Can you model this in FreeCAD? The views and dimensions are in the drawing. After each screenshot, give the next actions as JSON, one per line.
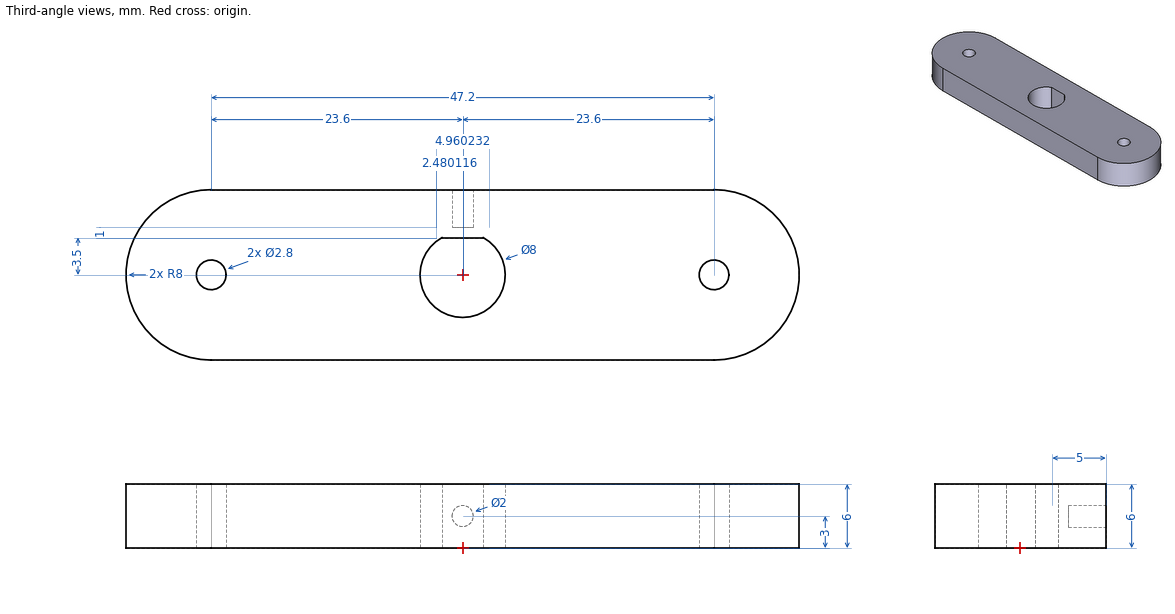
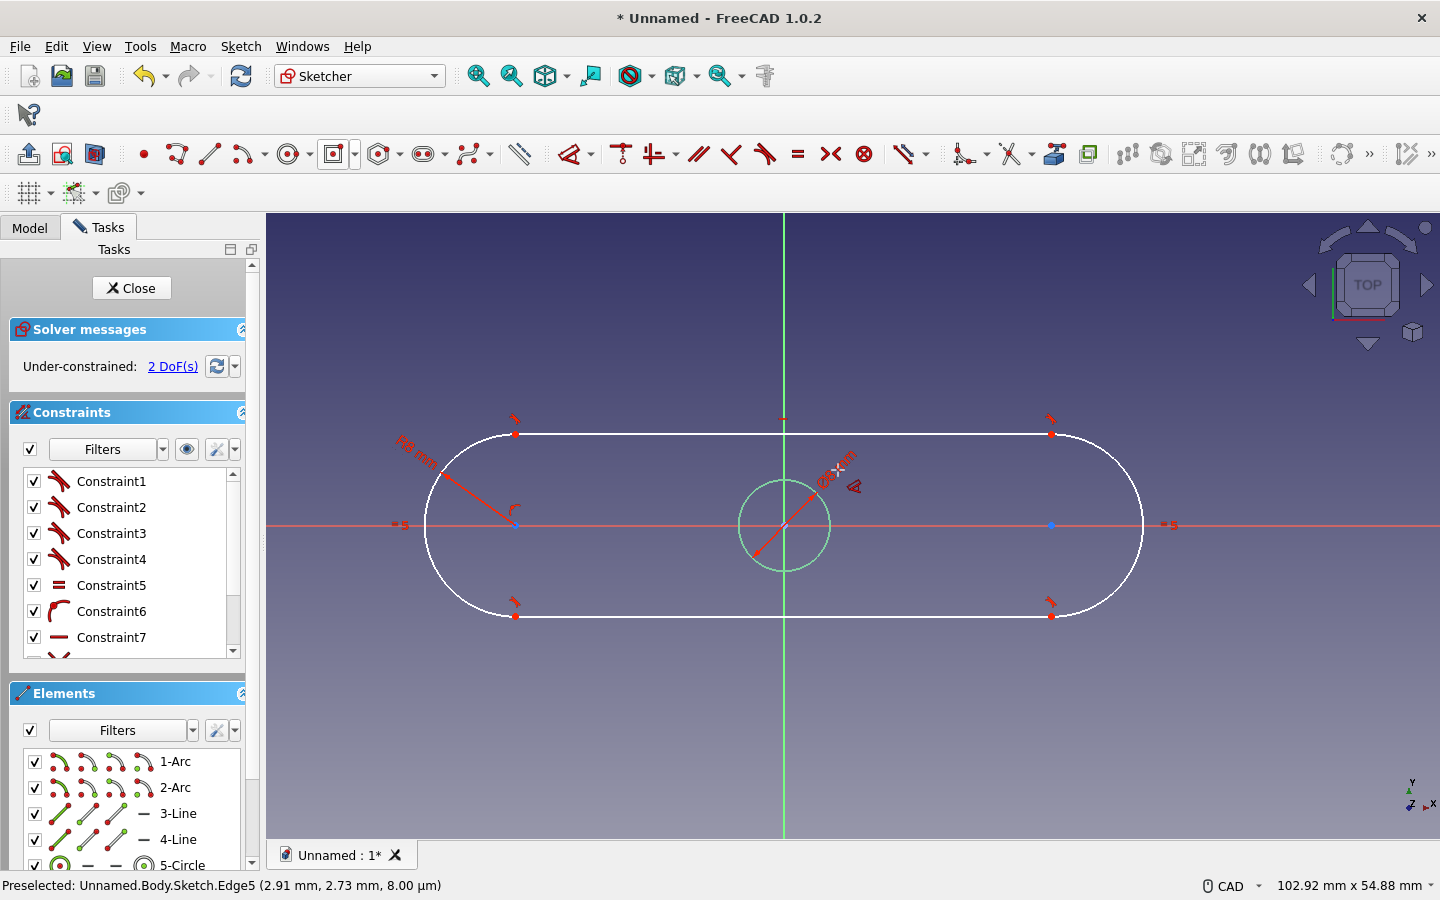
{"action": "left_click", "coordinate": [677, 434]}
{"action": "left_click", "coordinate": [661, 400]}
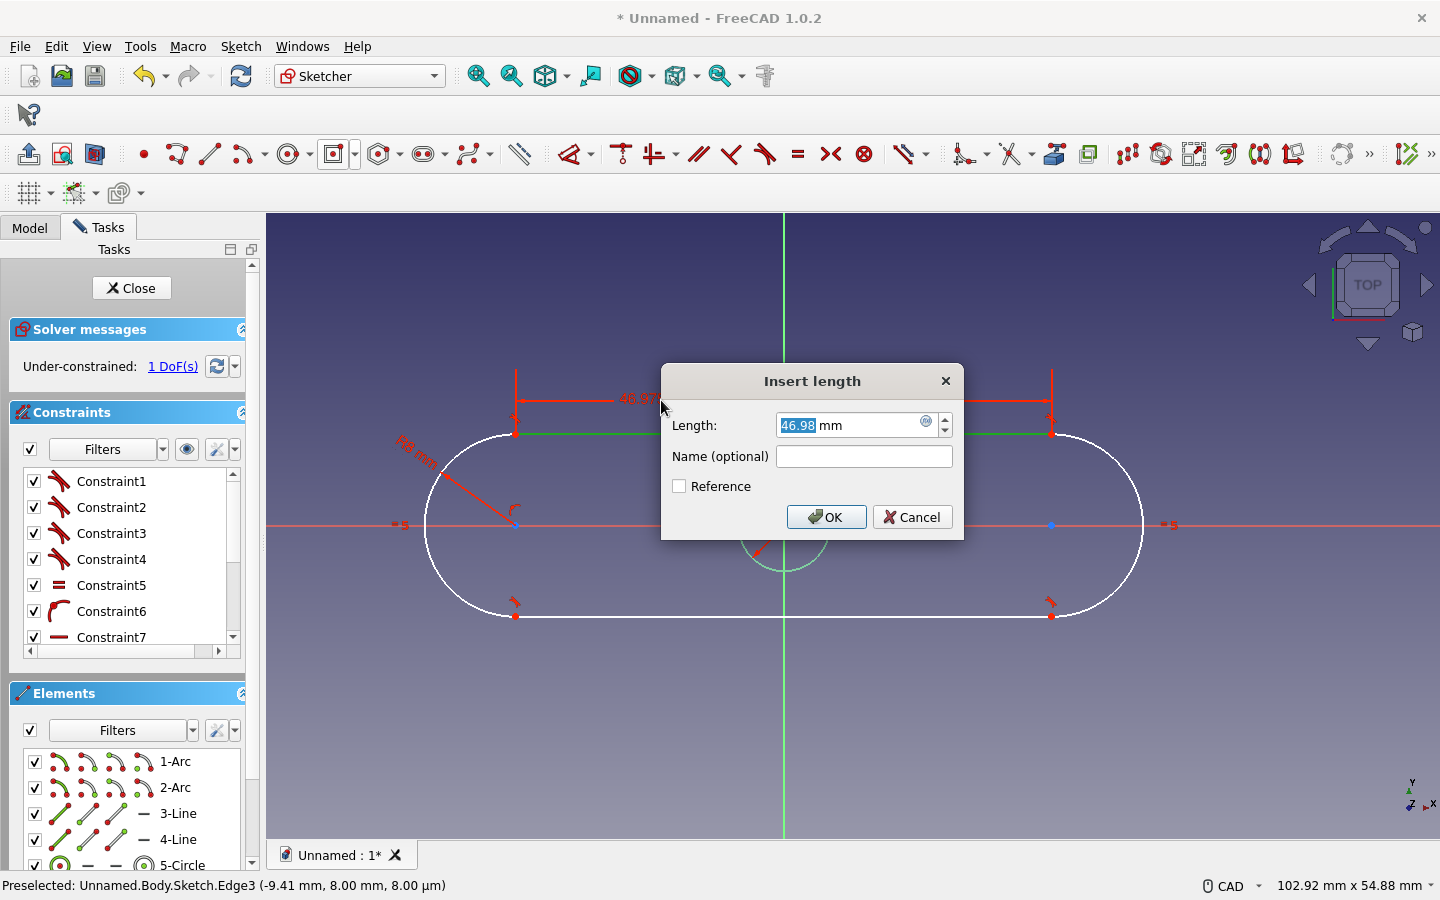
{"action": "type", "text": "47.2"}
{"action": "key", "text": "Return"}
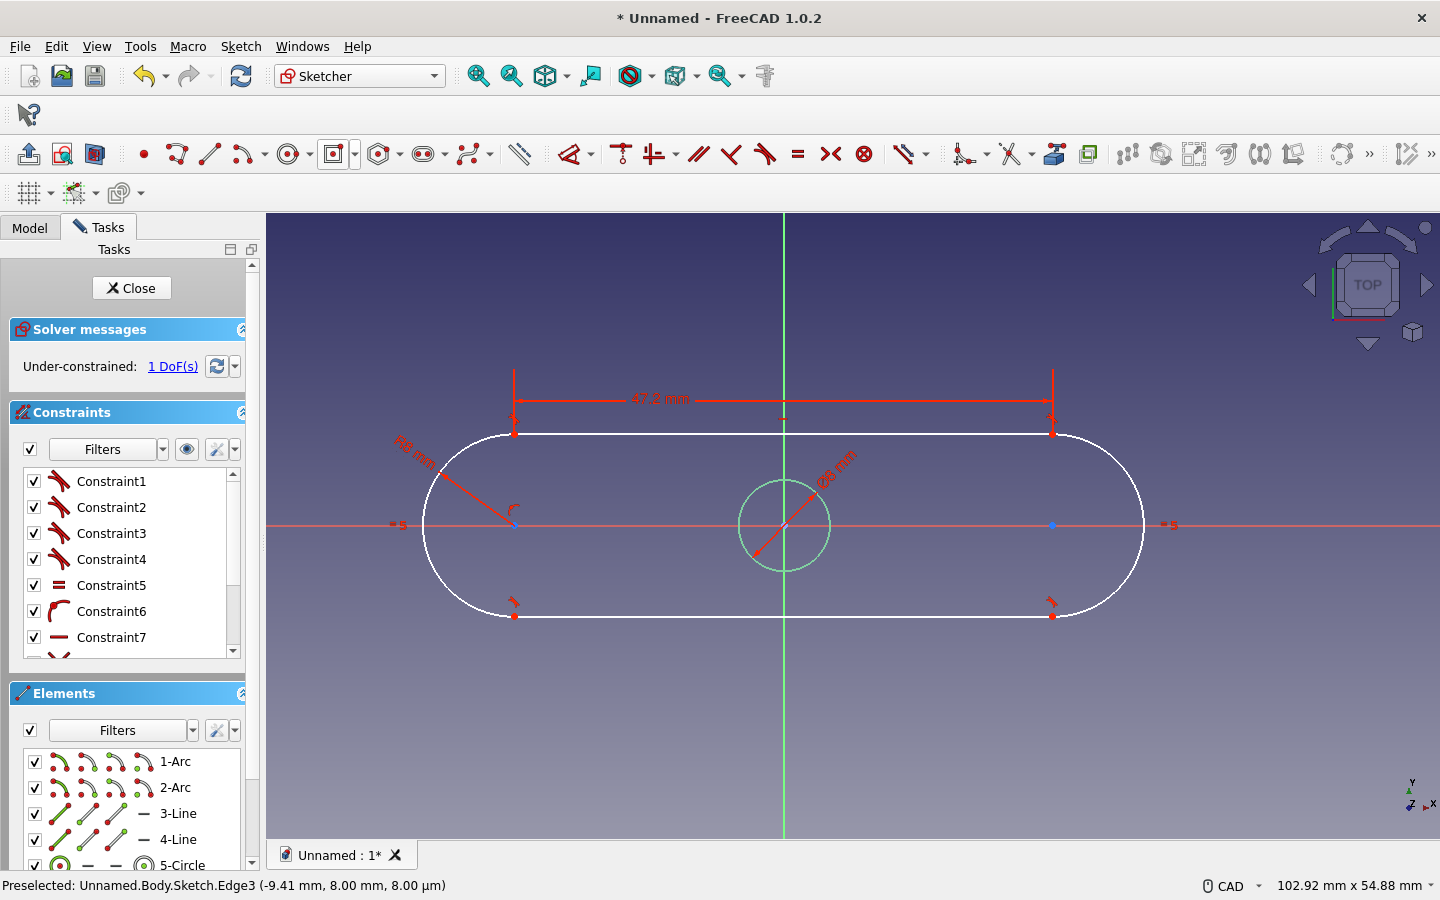
{"action": "left_click", "coordinate": [514, 434]}
{"action": "left_click", "coordinate": [587, 400]}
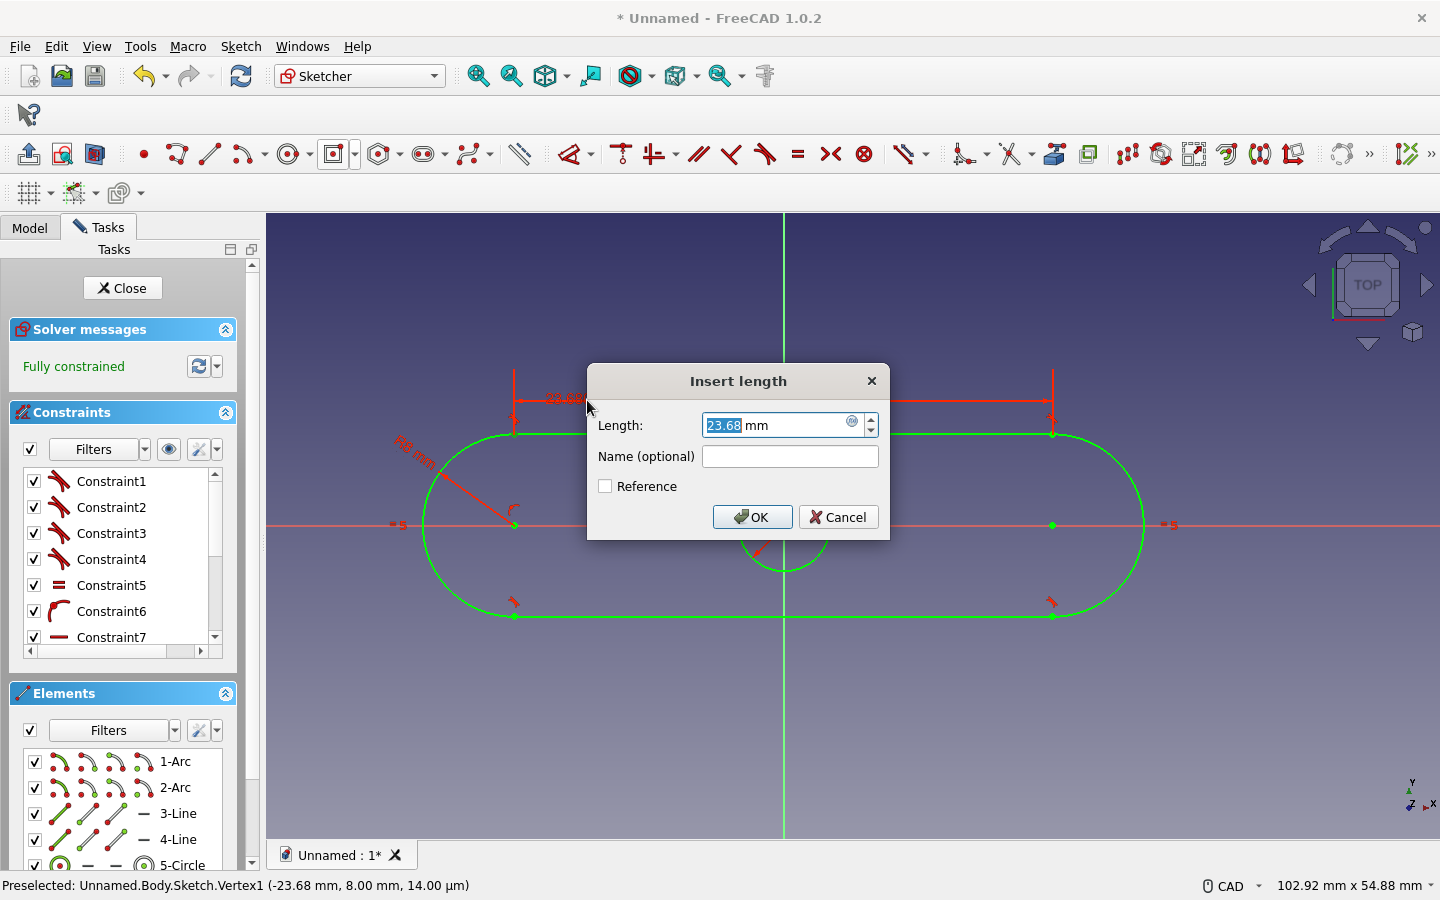
{"action": "type", "text": "23.6"}
{"action": "key", "text": "Return"}
{"action": "key", "text": "Escape"}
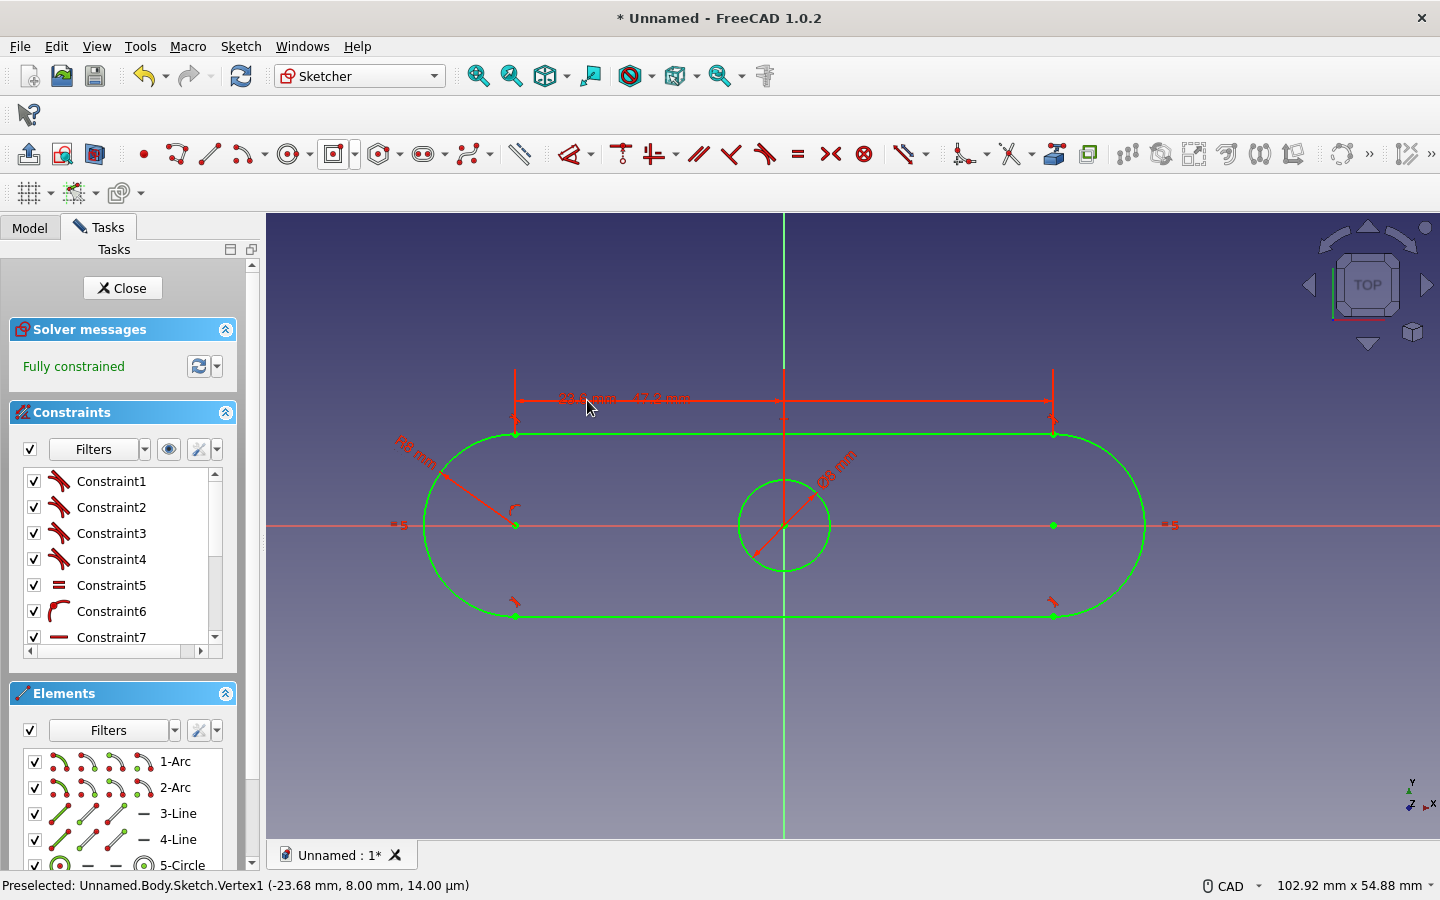
{"action": "left_click", "coordinate": [123, 288]}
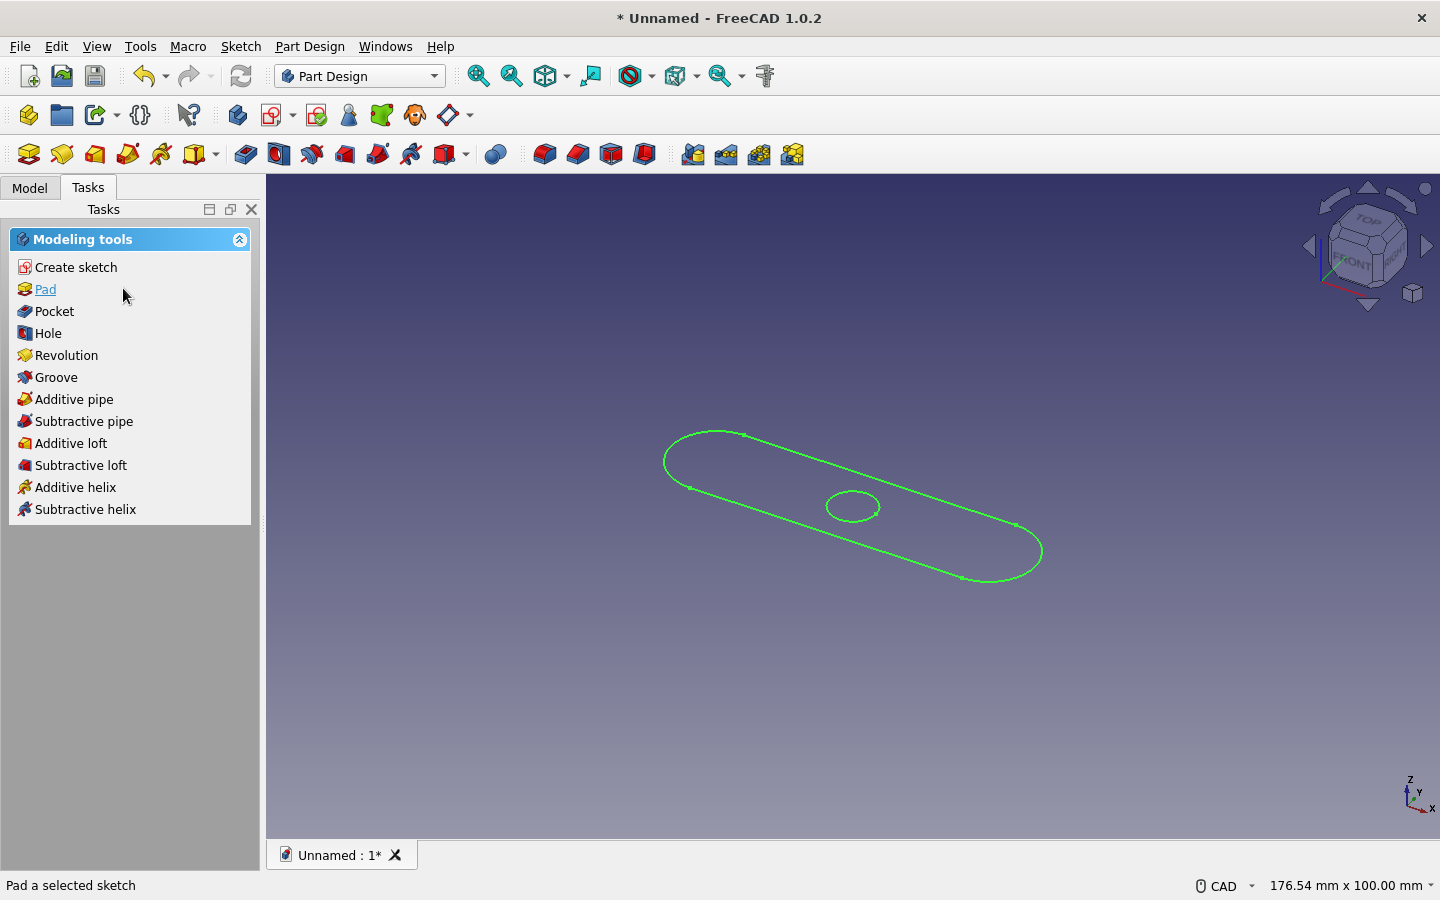
{"action": "left_click", "coordinate": [29, 154]}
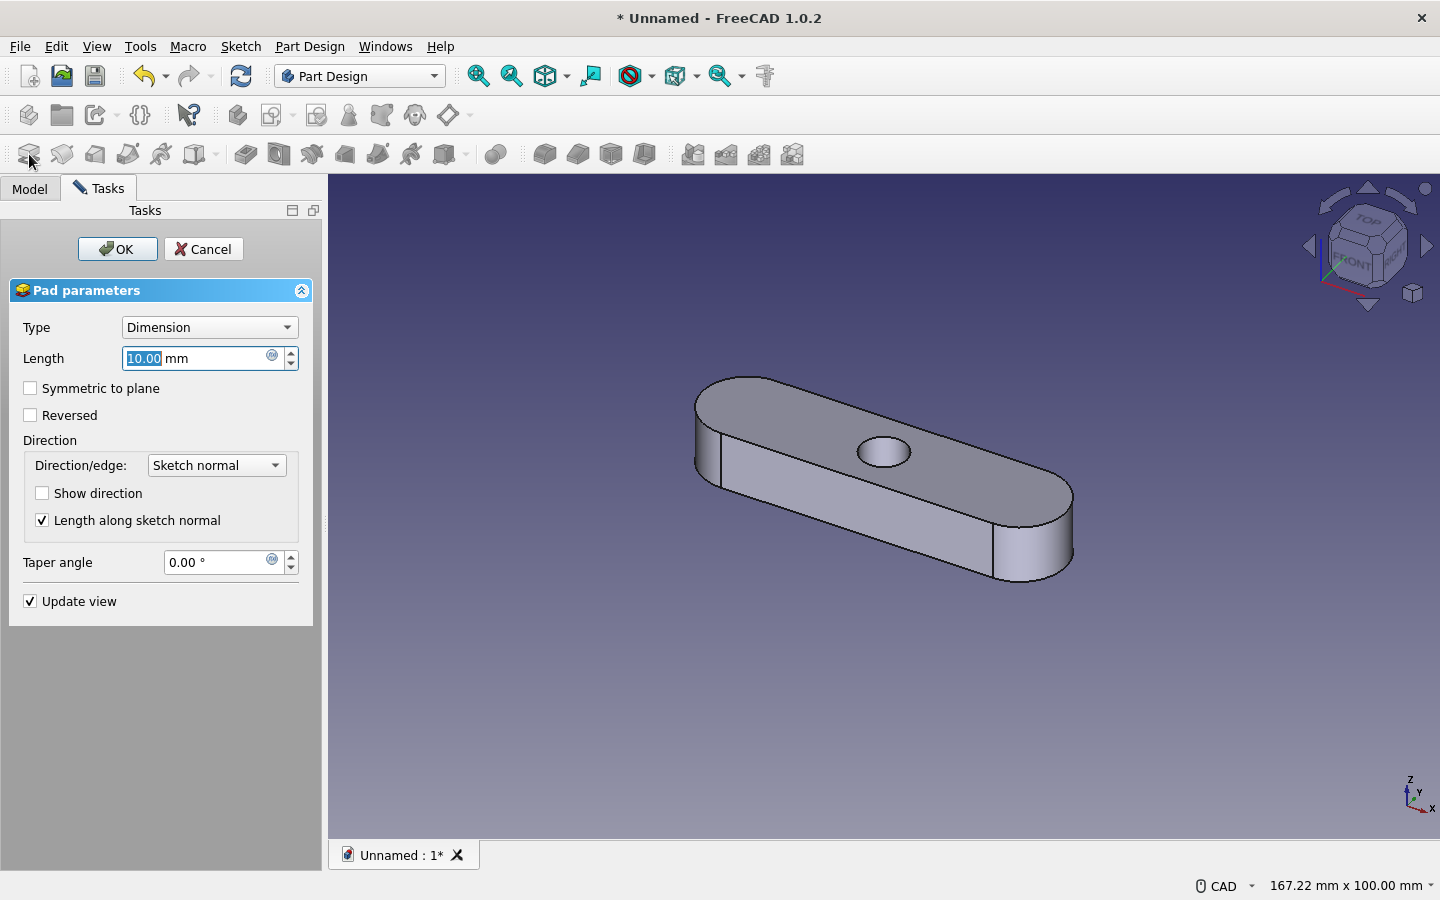
{"action": "type", "text": "6"}
{"action": "key", "text": "Tab"}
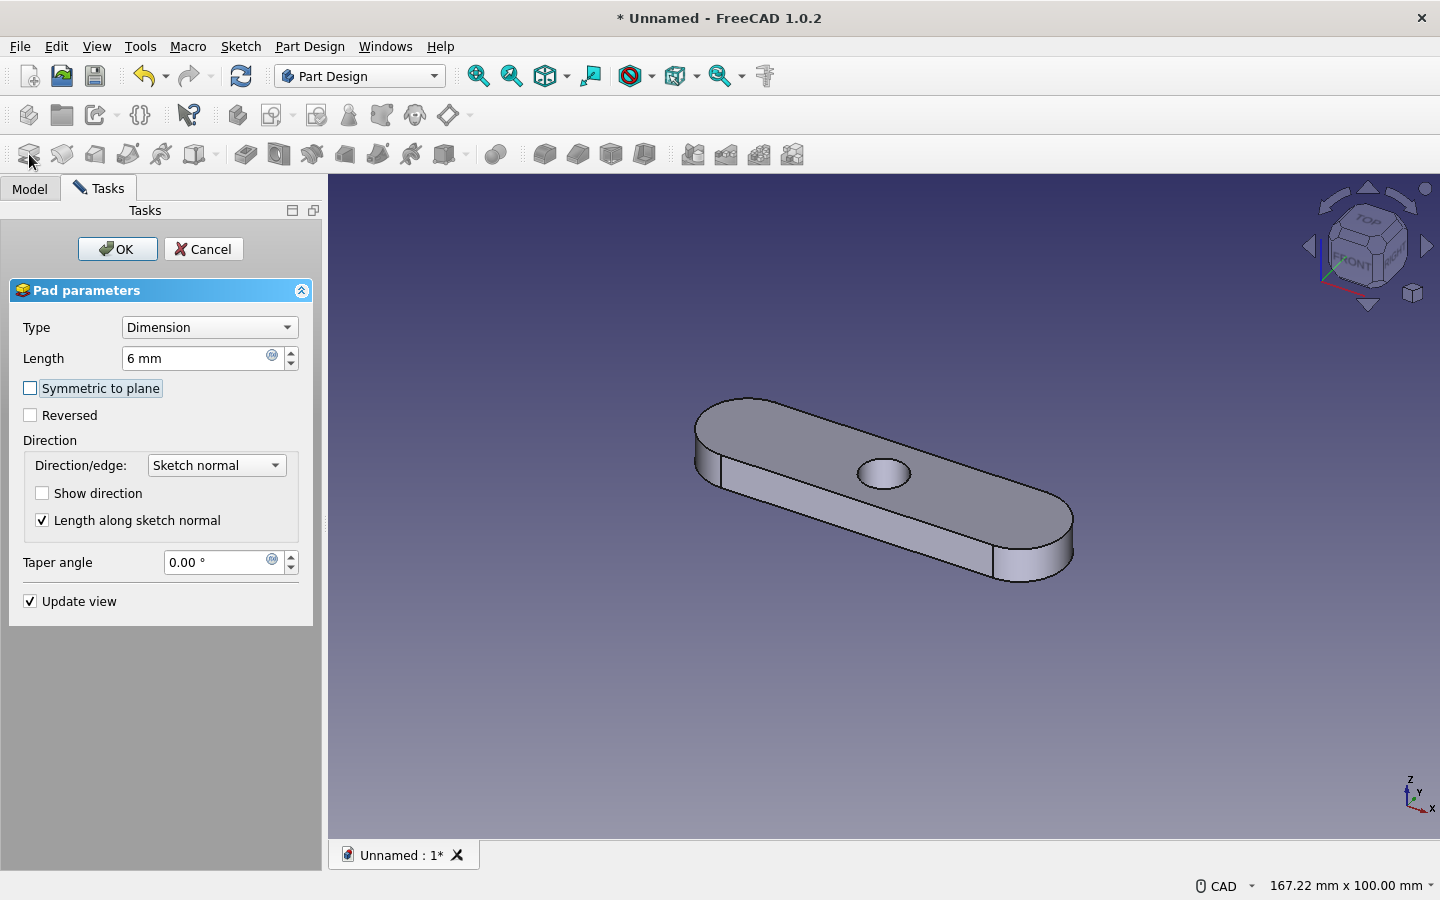
{"action": "left_click", "coordinate": [118, 249]}